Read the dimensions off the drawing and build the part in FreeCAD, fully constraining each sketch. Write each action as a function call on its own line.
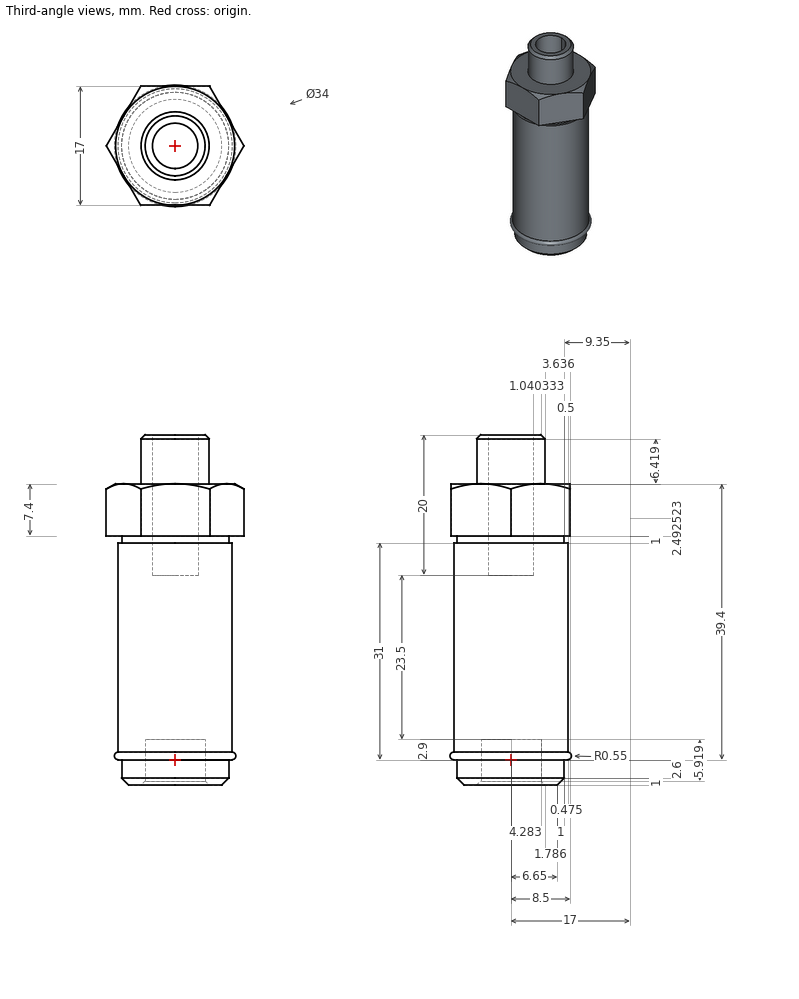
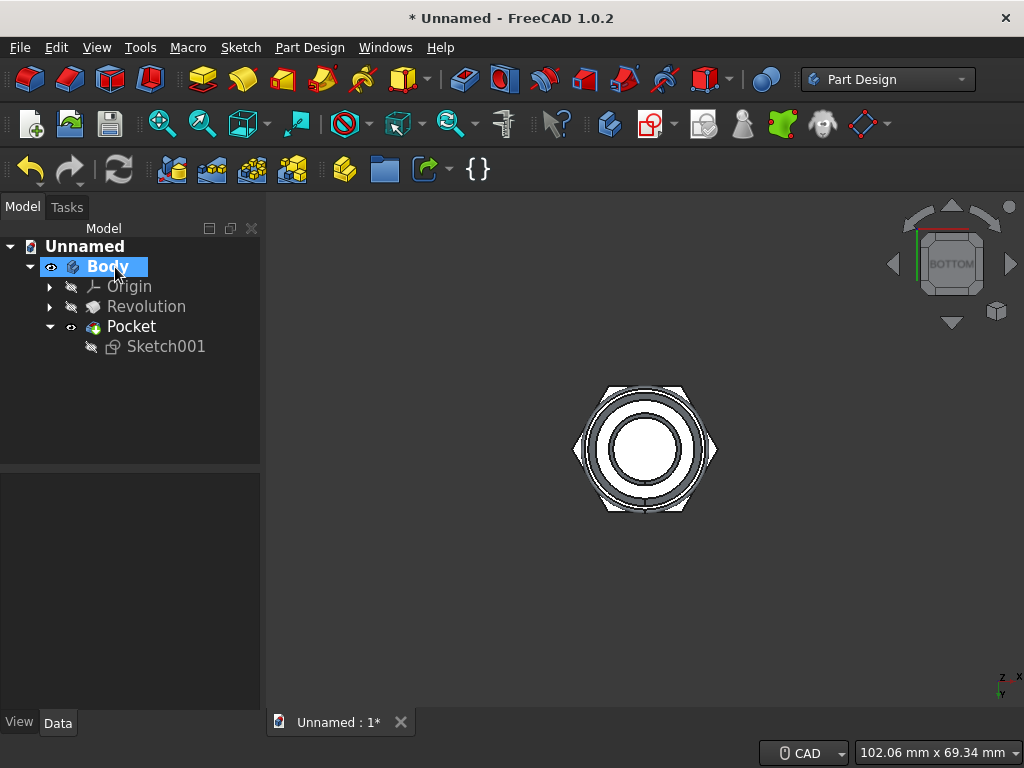
key(0)